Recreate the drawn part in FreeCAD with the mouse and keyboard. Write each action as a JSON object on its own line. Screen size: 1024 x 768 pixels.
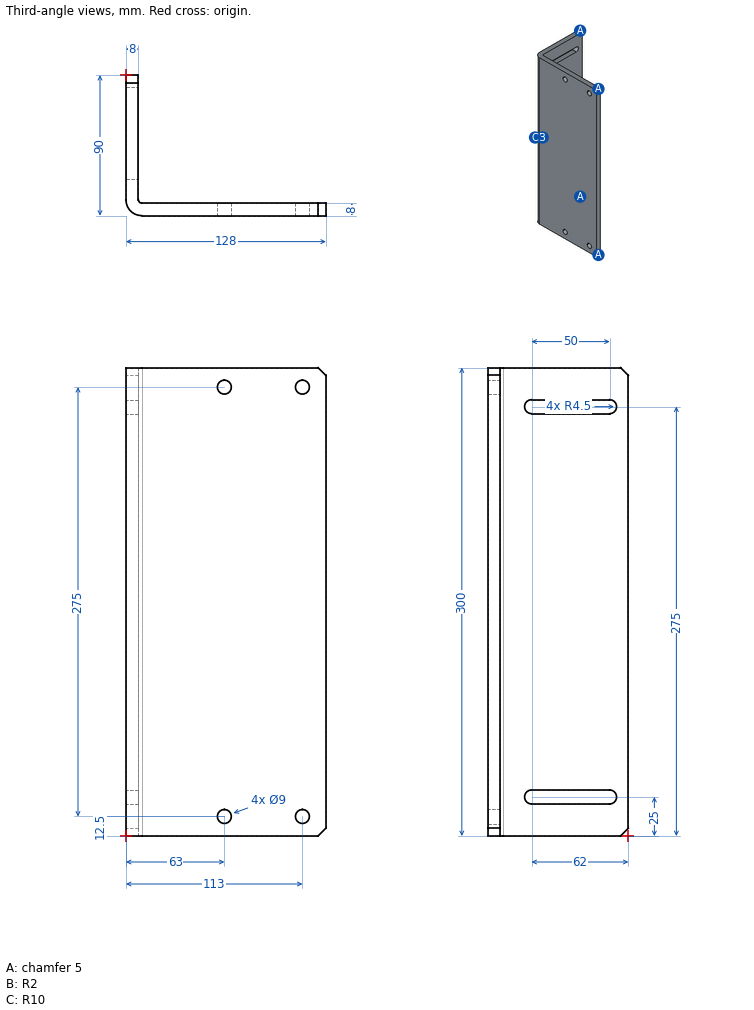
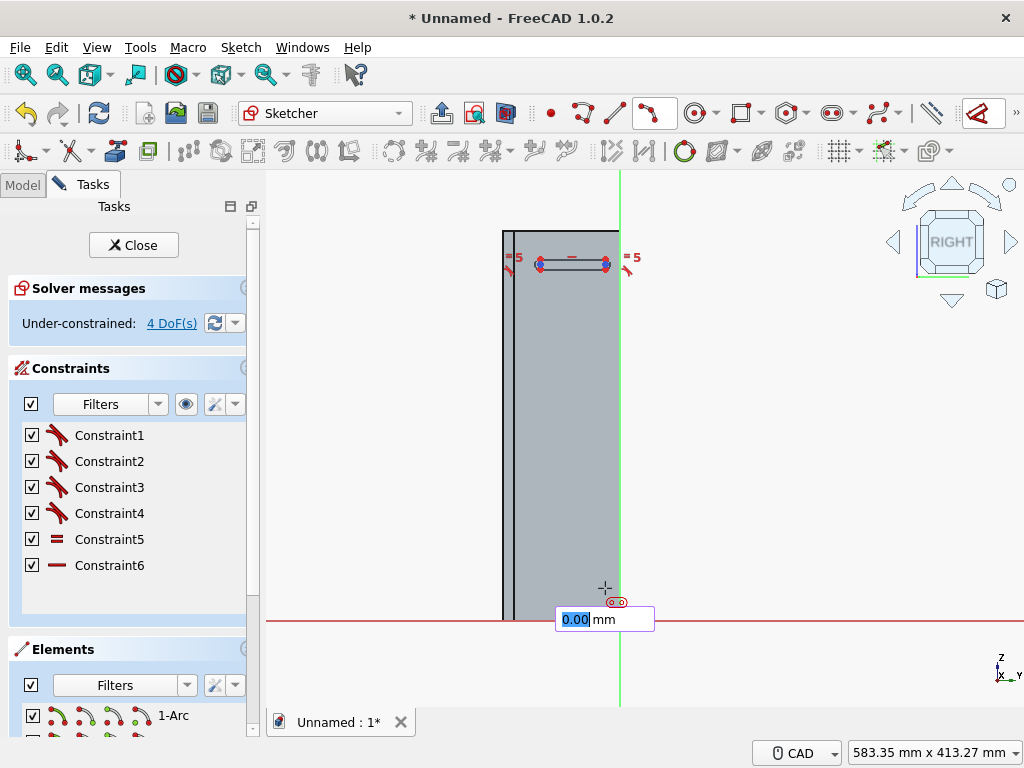
{"action": "scroll", "coordinate": [572, 583], "scroll_direction": "up", "scroll_amount": 5}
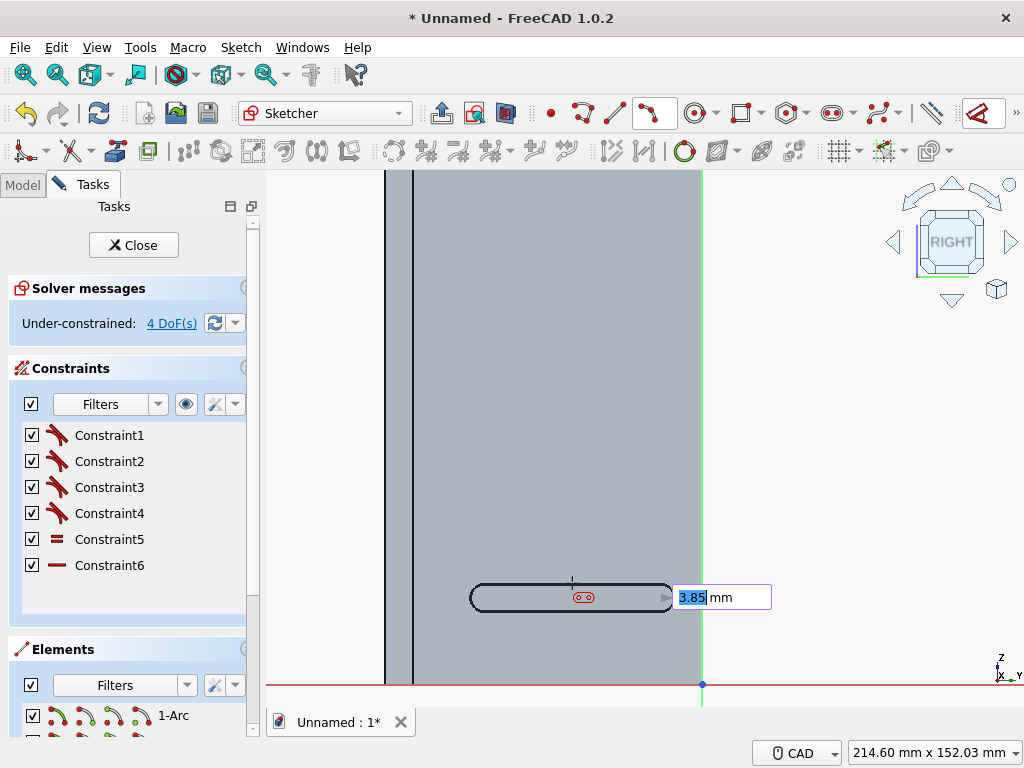
{"action": "left_click", "coordinate": [572, 581]}
{"action": "key", "text": "Escape"}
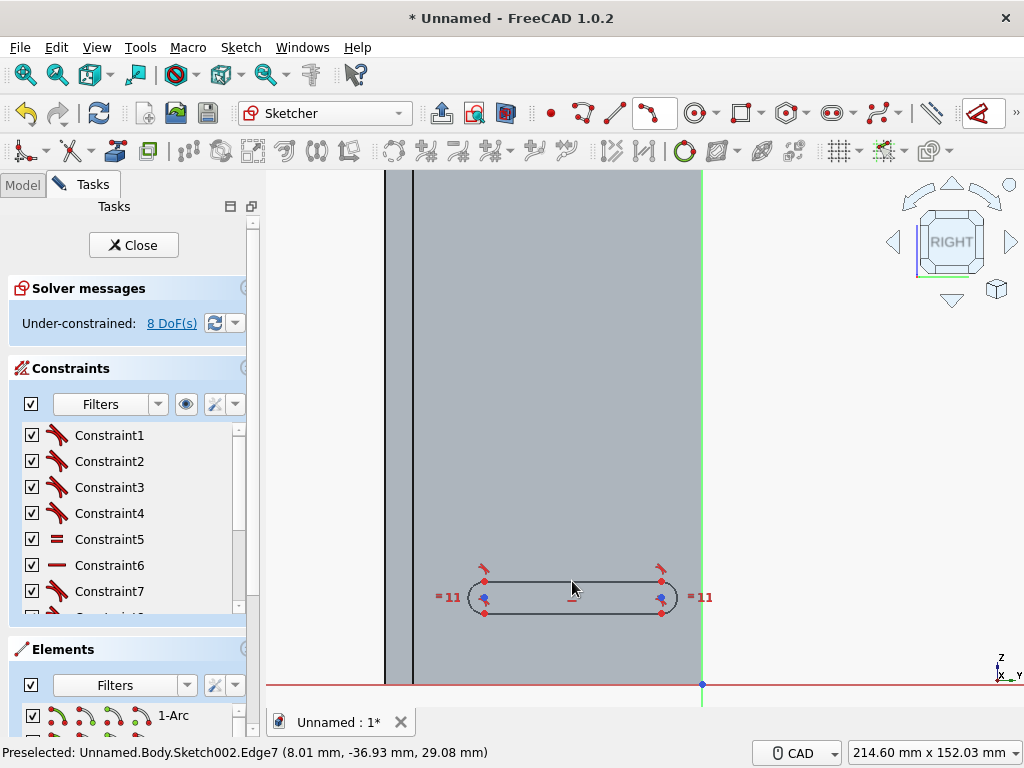
{"action": "scroll", "coordinate": [572, 582], "scroll_direction": "down", "scroll_amount": 5}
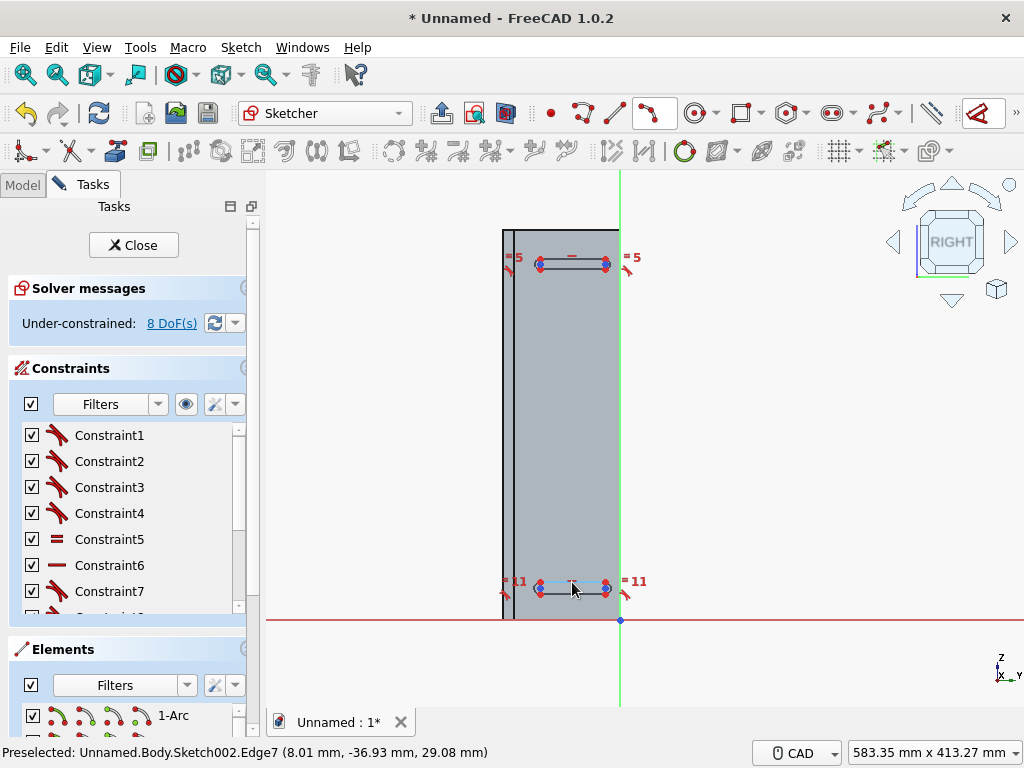
{"action": "scroll", "coordinate": [536, 261], "scroll_direction": "up", "scroll_amount": 6}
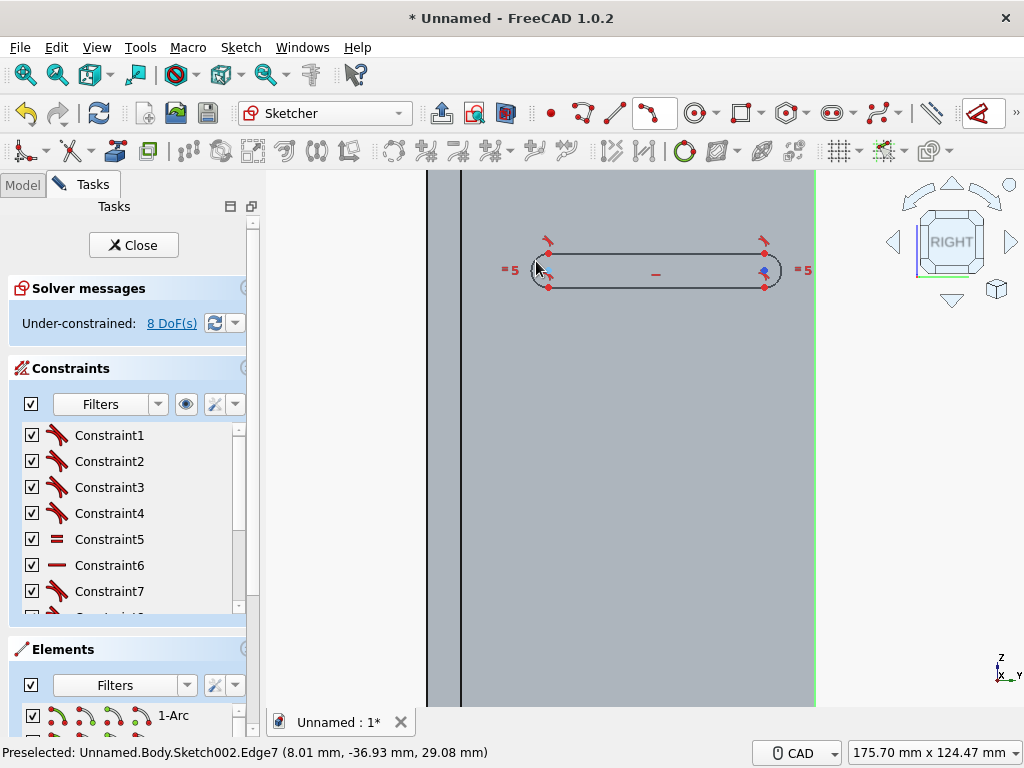
{"action": "left_click", "coordinate": [535, 261]}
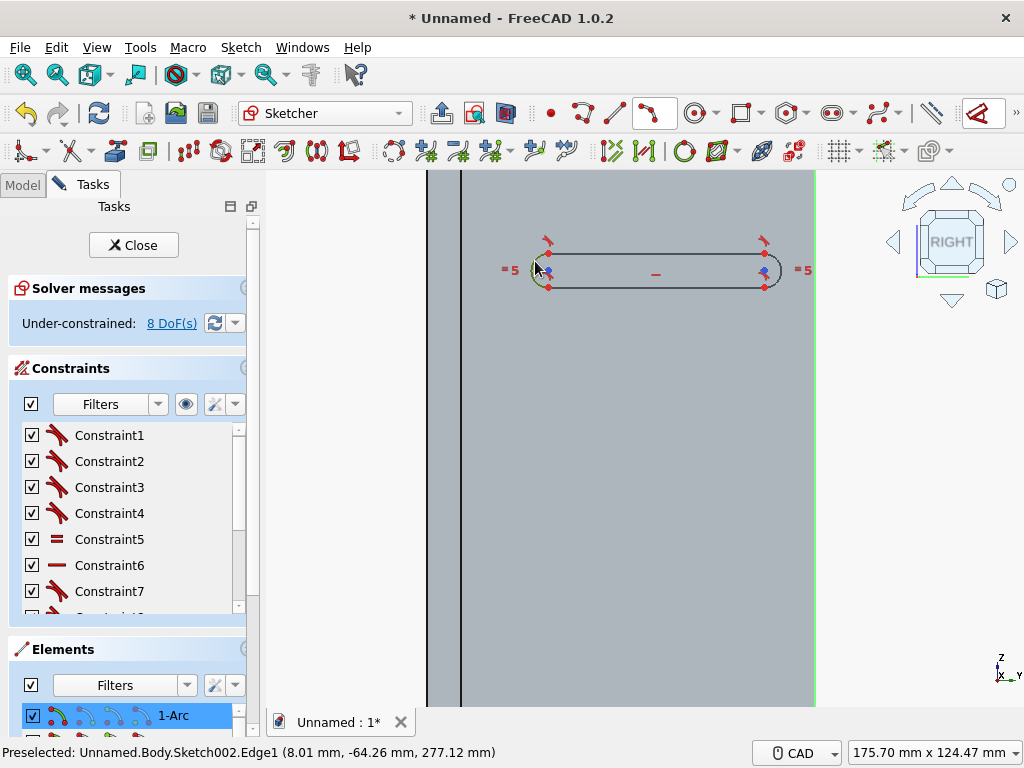
{"action": "scroll", "coordinate": [536, 261], "scroll_direction": "down", "scroll_amount": 6}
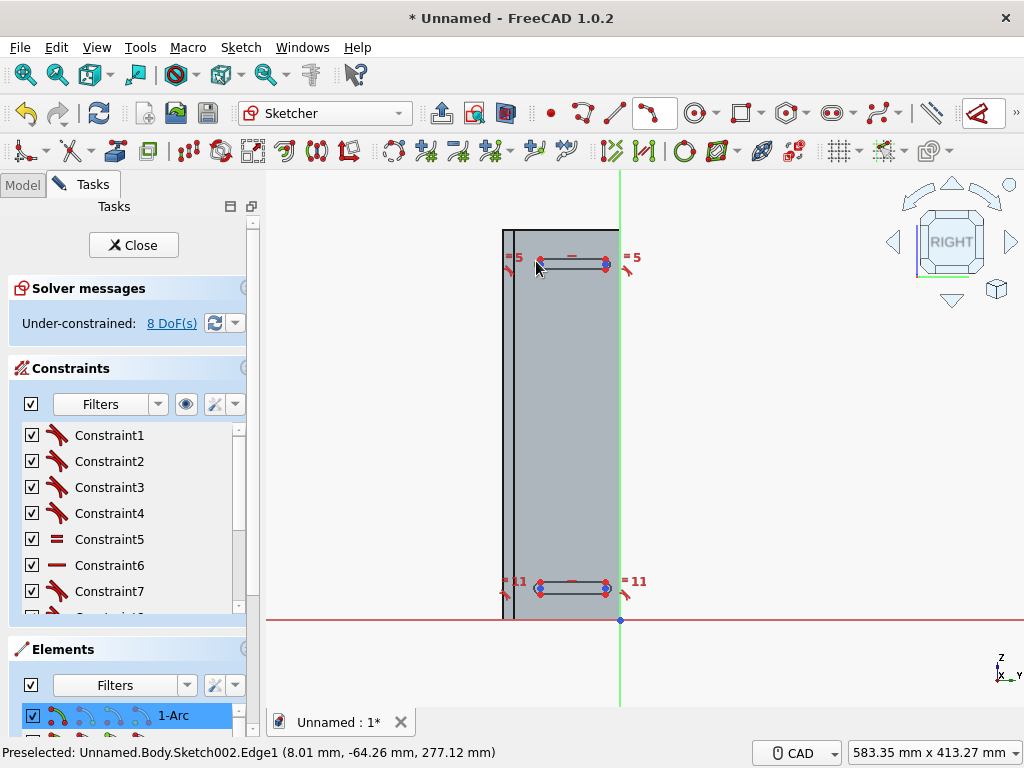
{"action": "scroll", "coordinate": [535, 585], "scroll_direction": "up", "scroll_amount": 5}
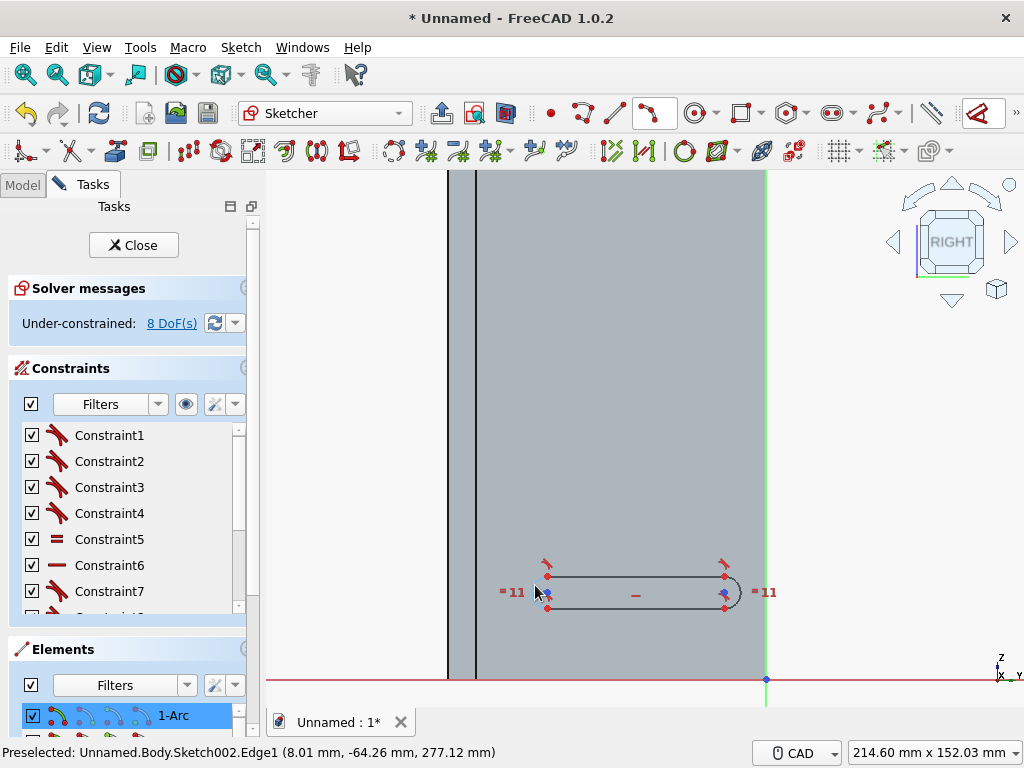
{"action": "left_click", "coordinate": [535, 583]}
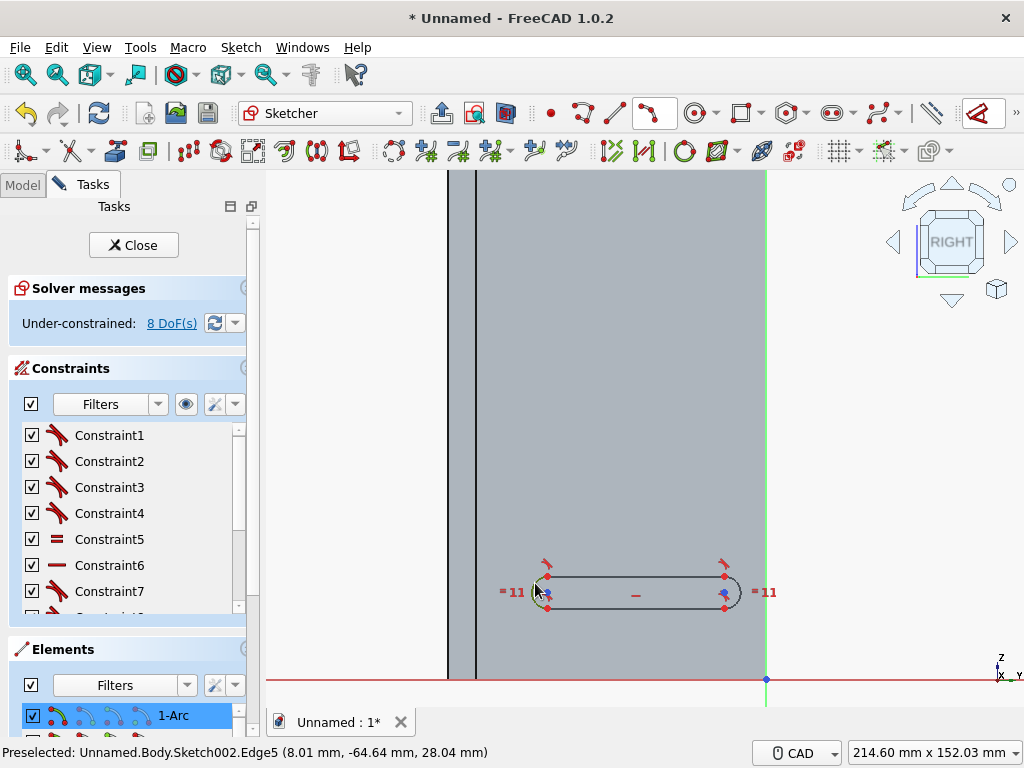
{"action": "key", "text": "e"}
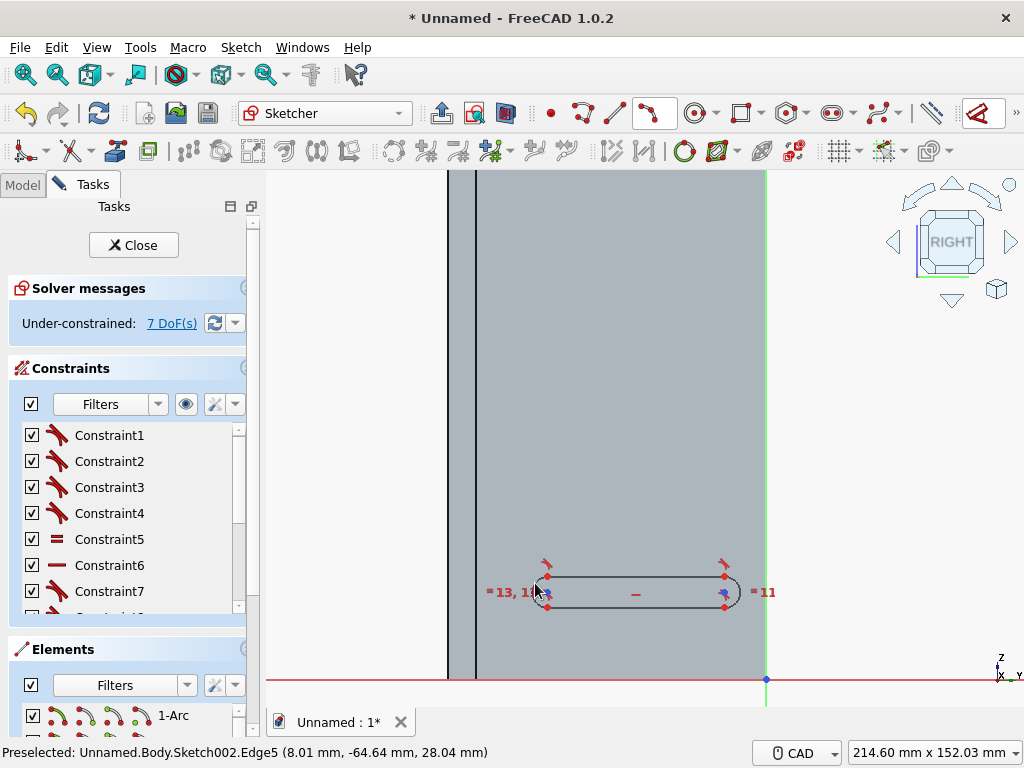
{"action": "left_click", "coordinate": [978, 114]}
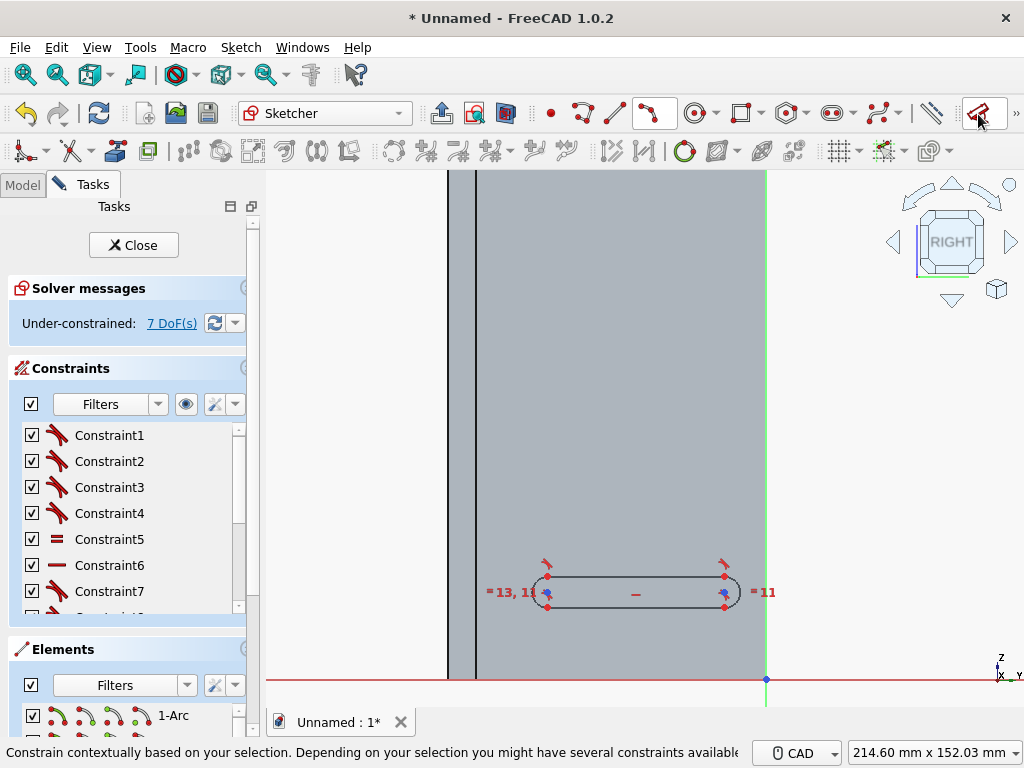
{"action": "scroll", "coordinate": [535, 585], "scroll_direction": "down", "scroll_amount": 5}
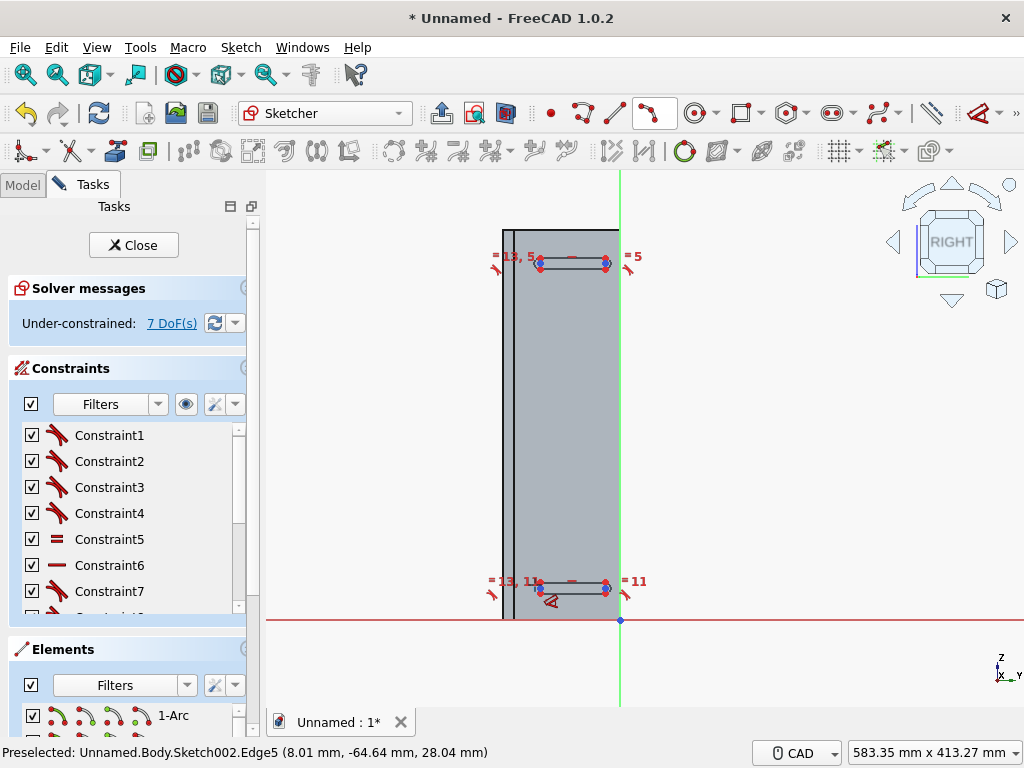
{"action": "scroll", "coordinate": [535, 260], "scroll_direction": "up", "scroll_amount": 10}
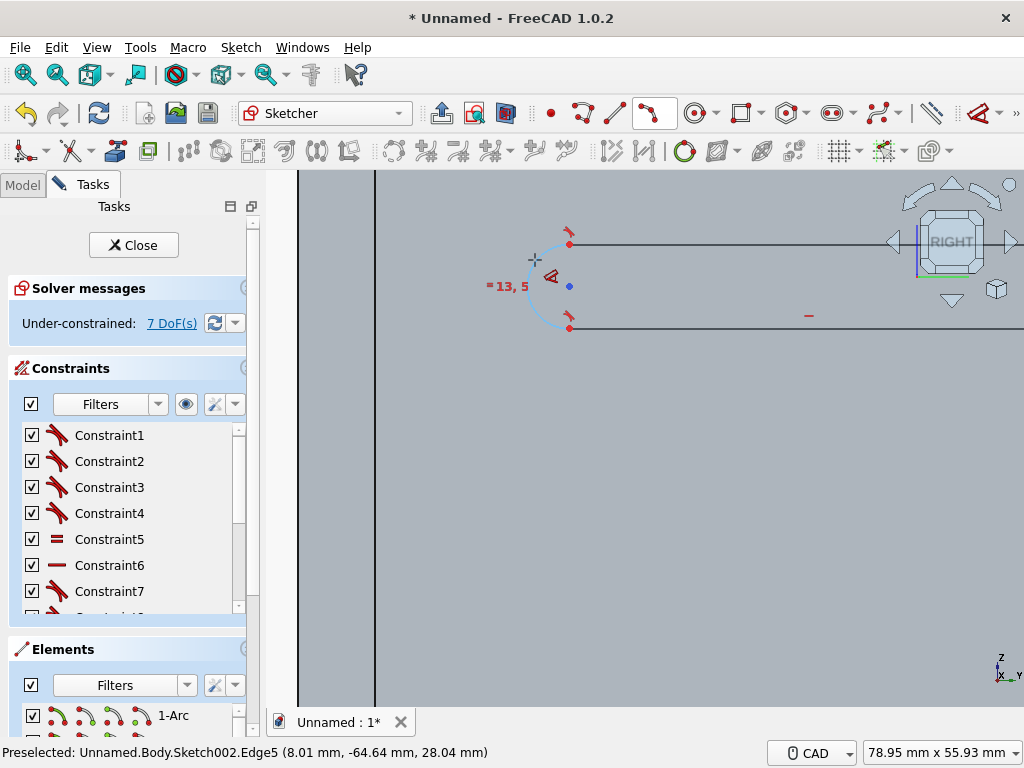
{"action": "left_click", "coordinate": [536, 262]}
{"action": "left_click", "coordinate": [510, 243]}